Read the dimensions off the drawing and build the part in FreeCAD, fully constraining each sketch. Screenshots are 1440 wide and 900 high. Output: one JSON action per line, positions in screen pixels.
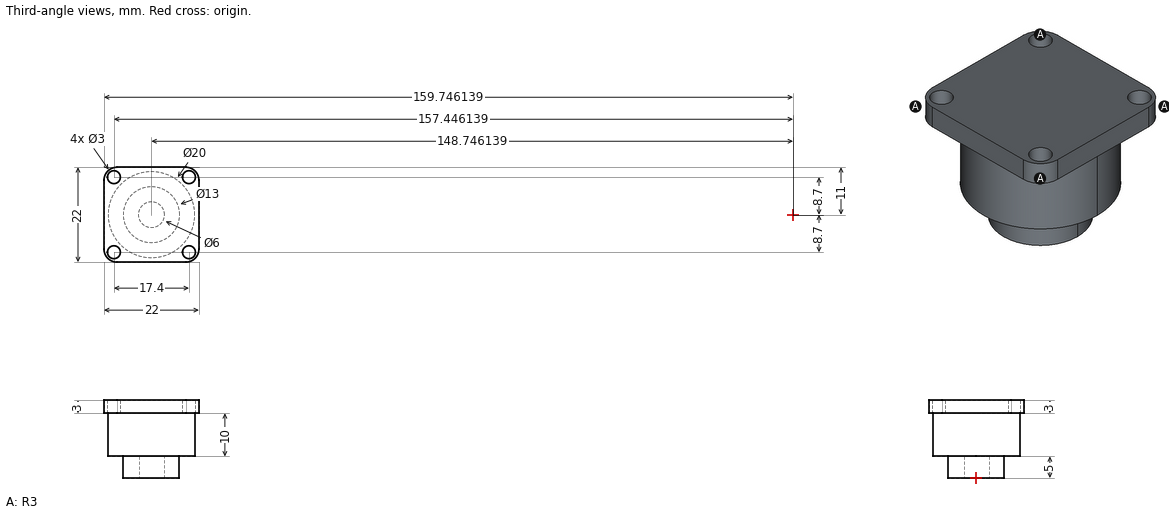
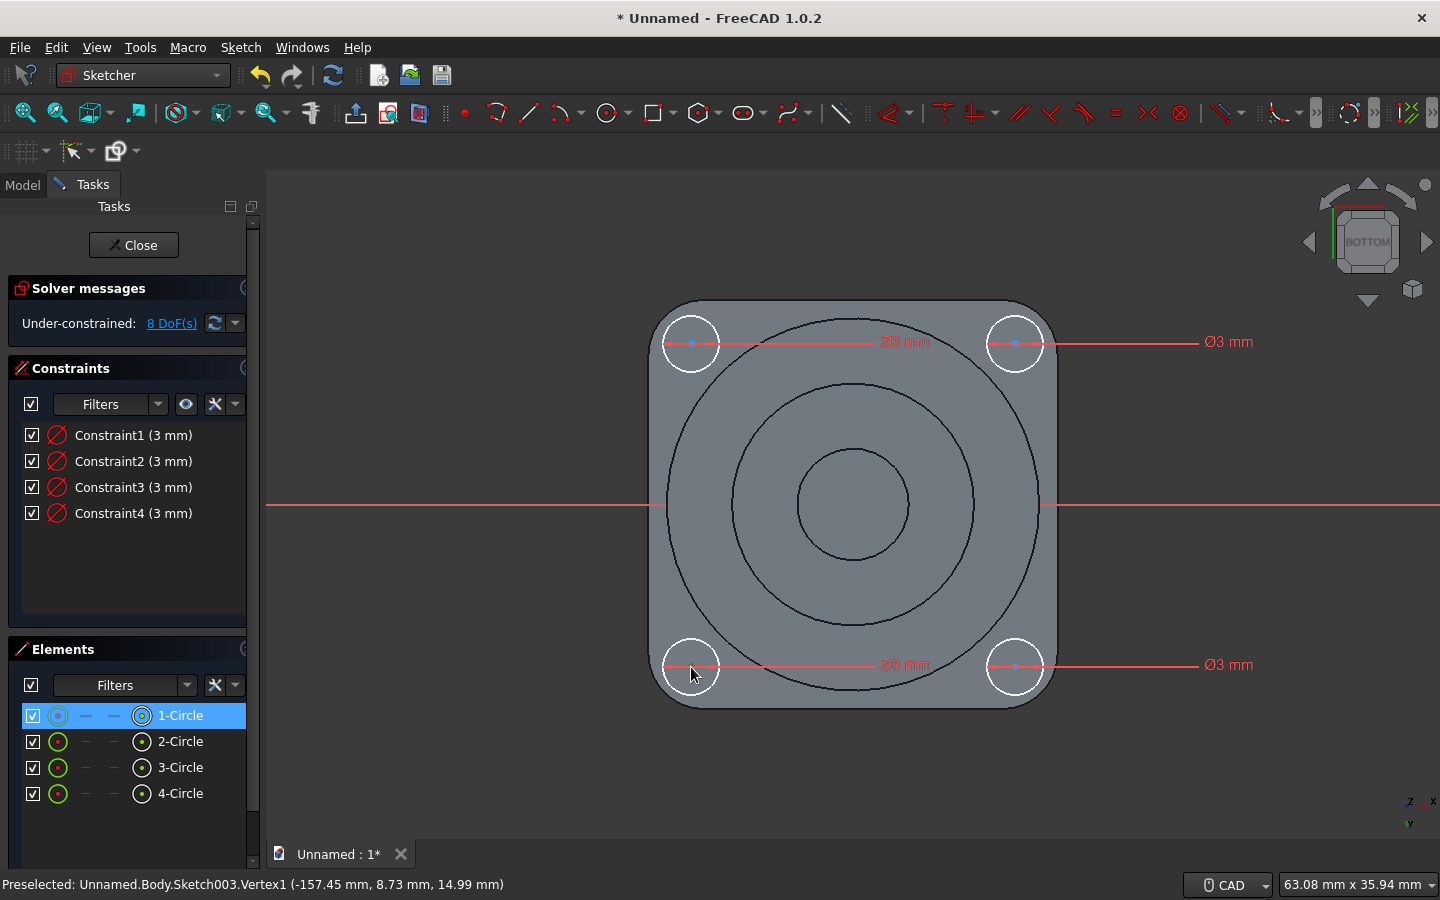
{"action": "left_click", "coordinate": [691, 344]}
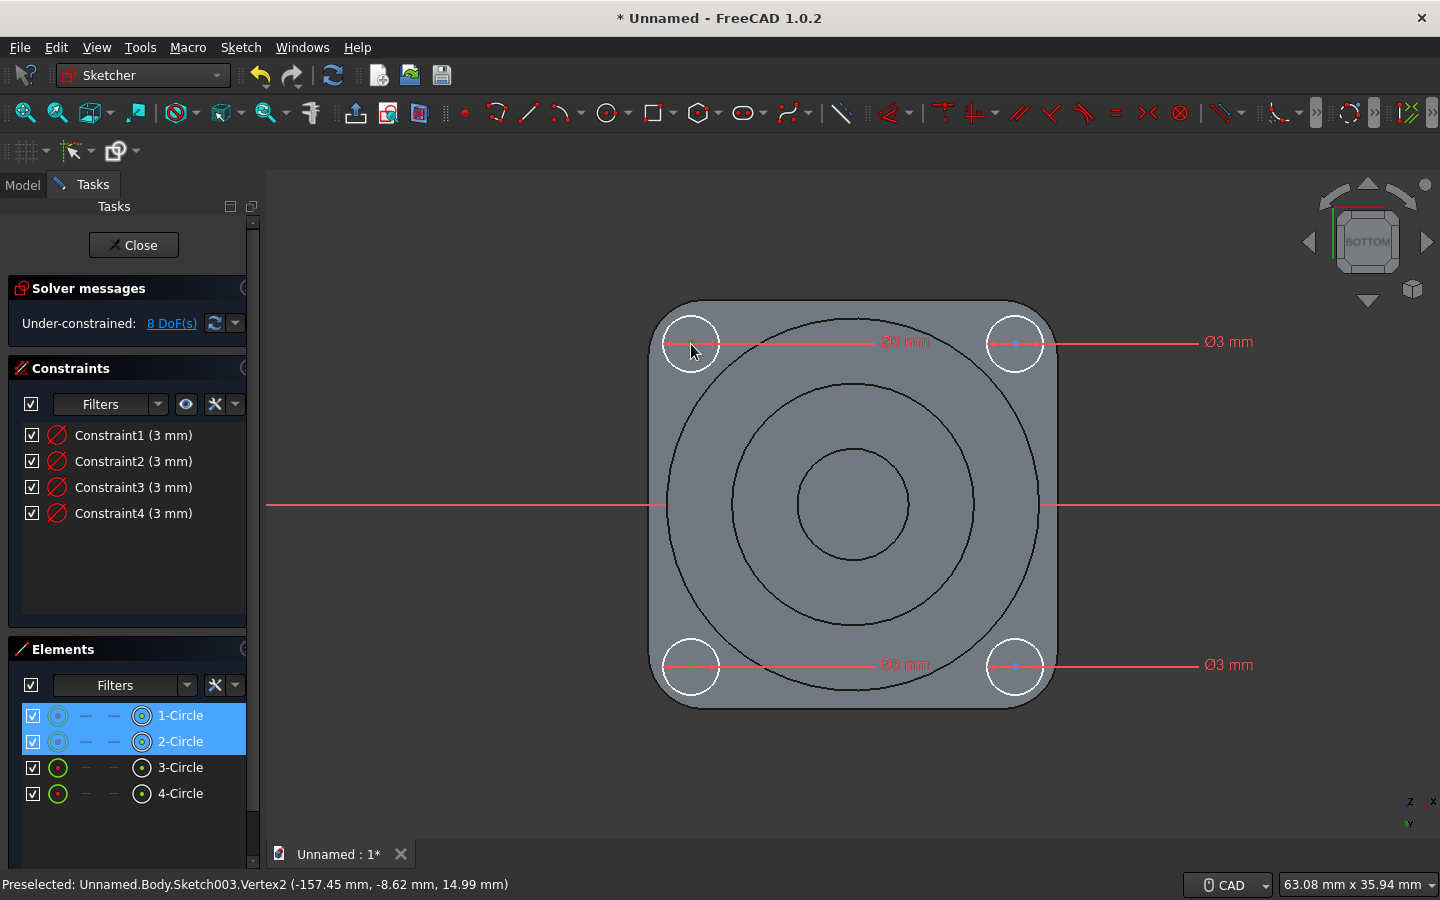
{"action": "key", "text": "v"}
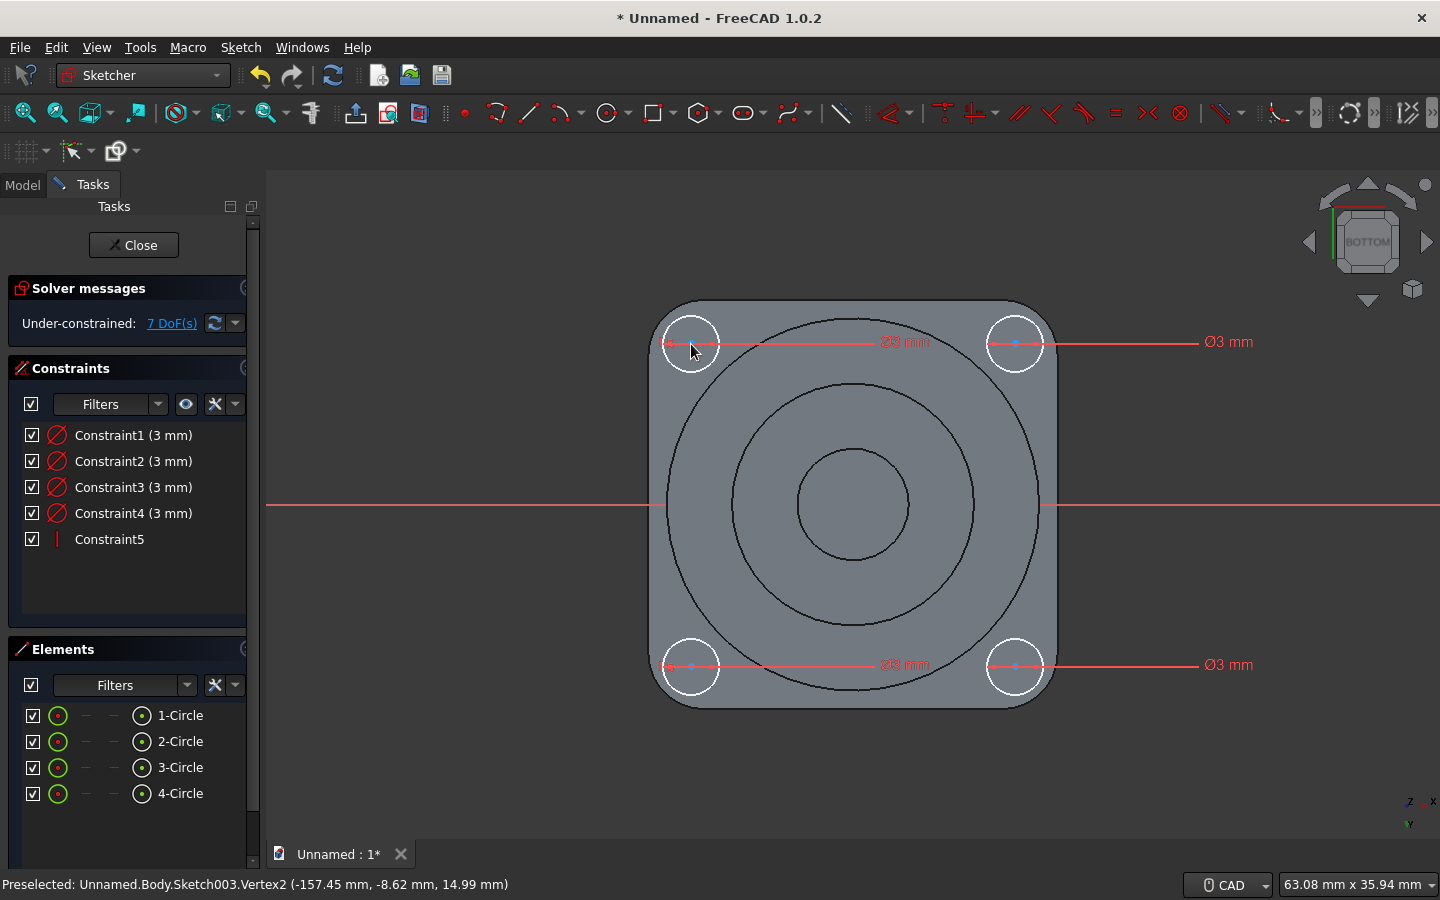
{"action": "left_click", "coordinate": [691, 344]}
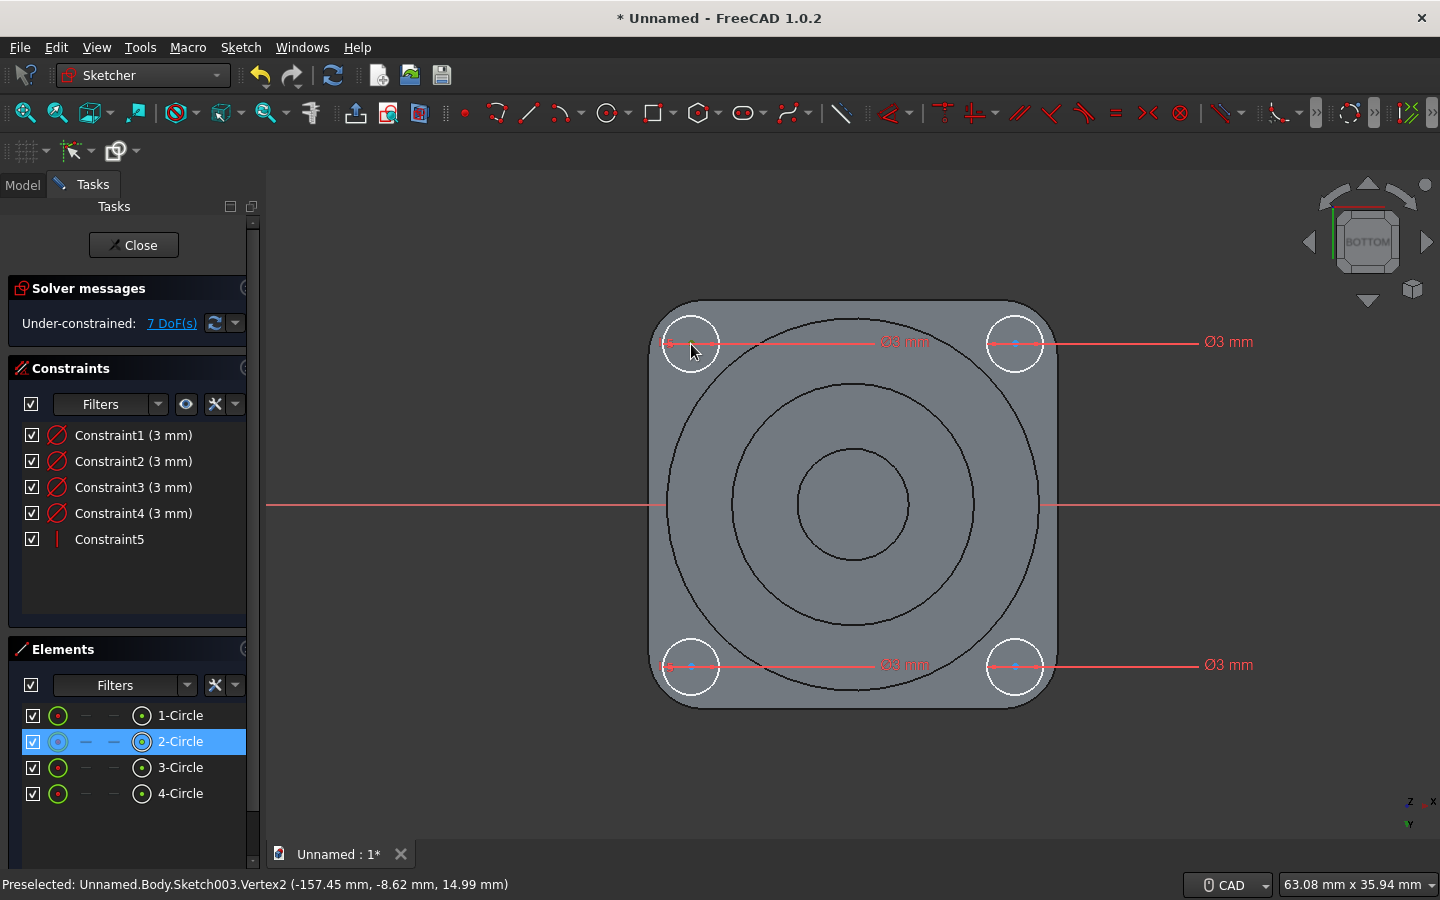
{"action": "left_click", "coordinate": [1015, 344]}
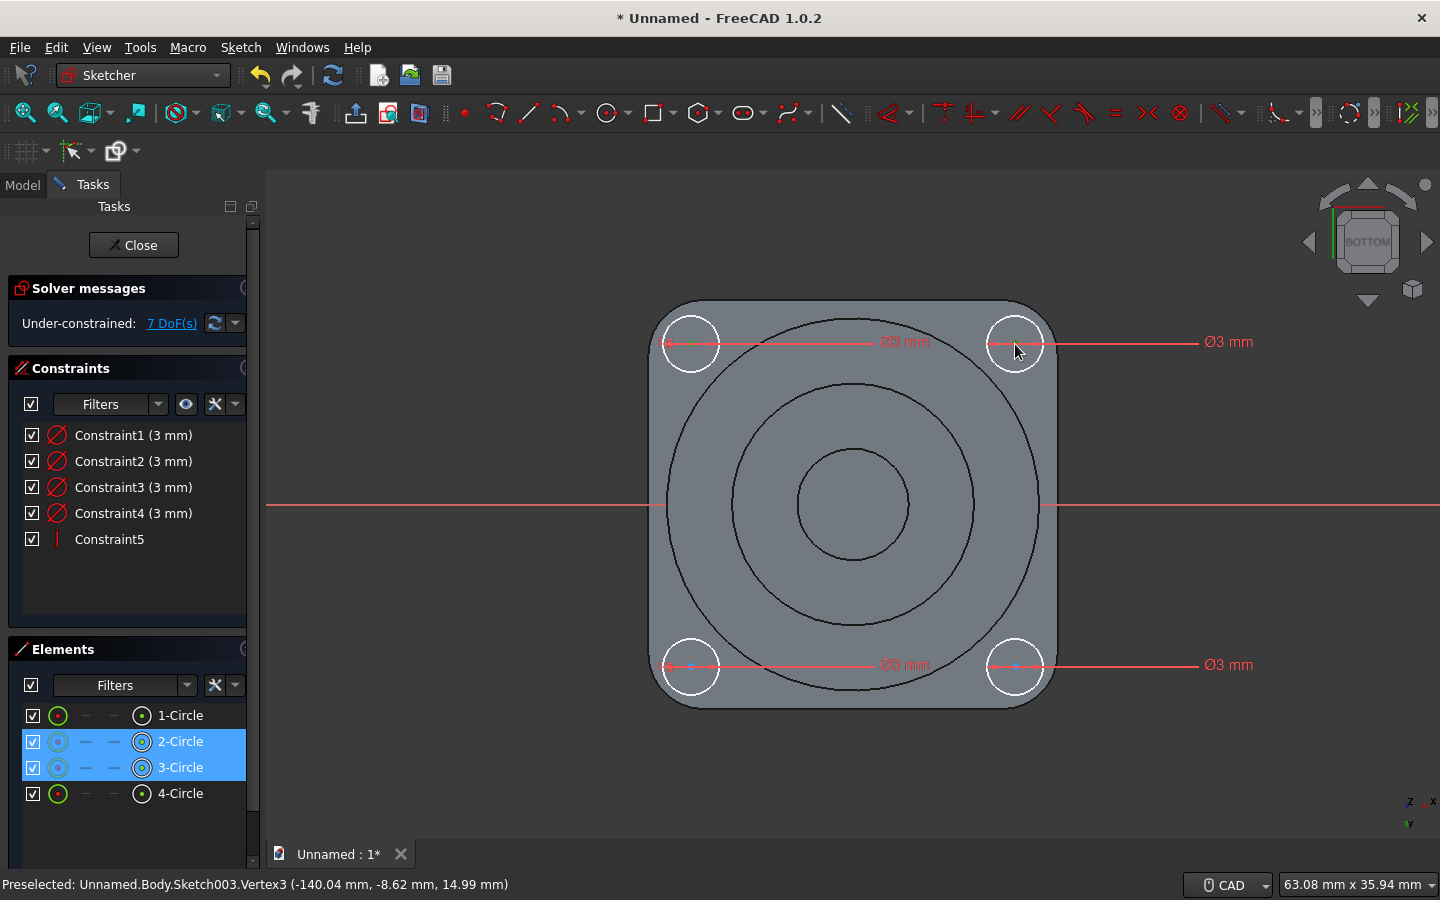
{"action": "left_click", "coordinate": [998, 114]}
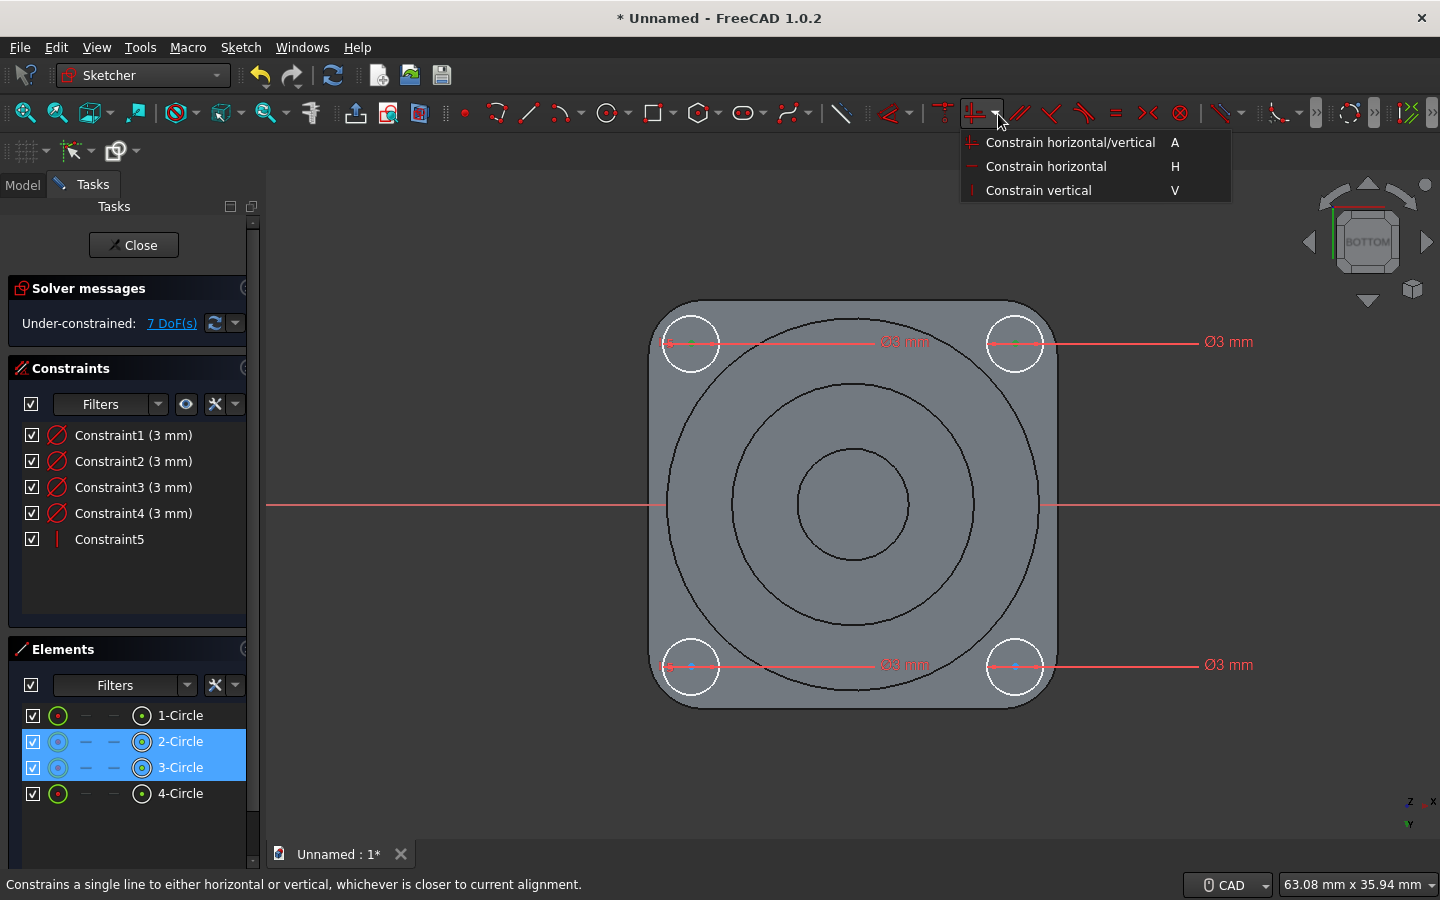
{"action": "left_click", "coordinate": [1096, 166]}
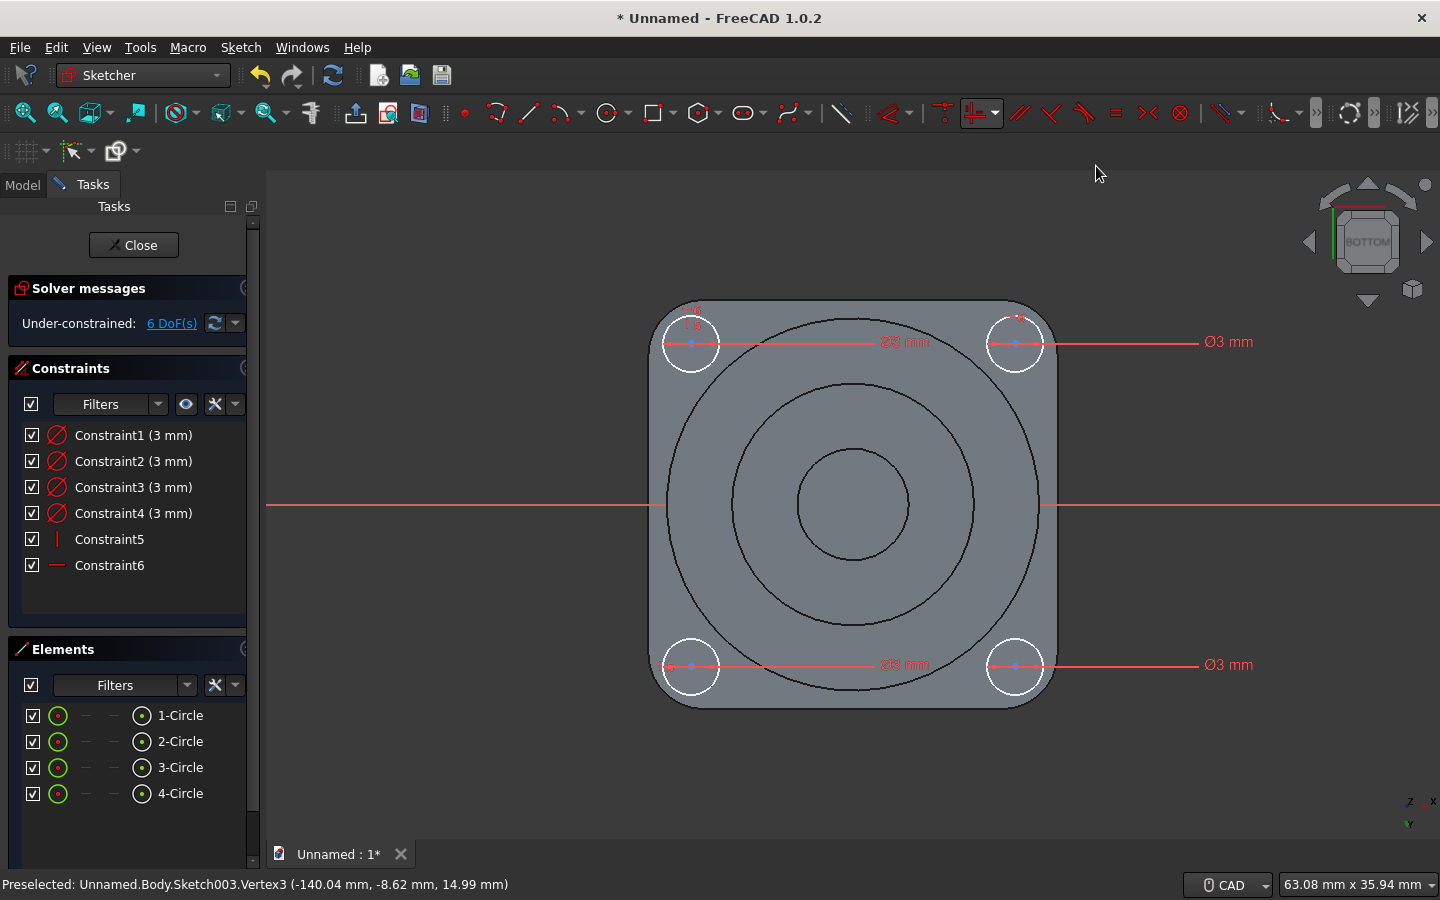
{"action": "left_click", "coordinate": [1015, 344]}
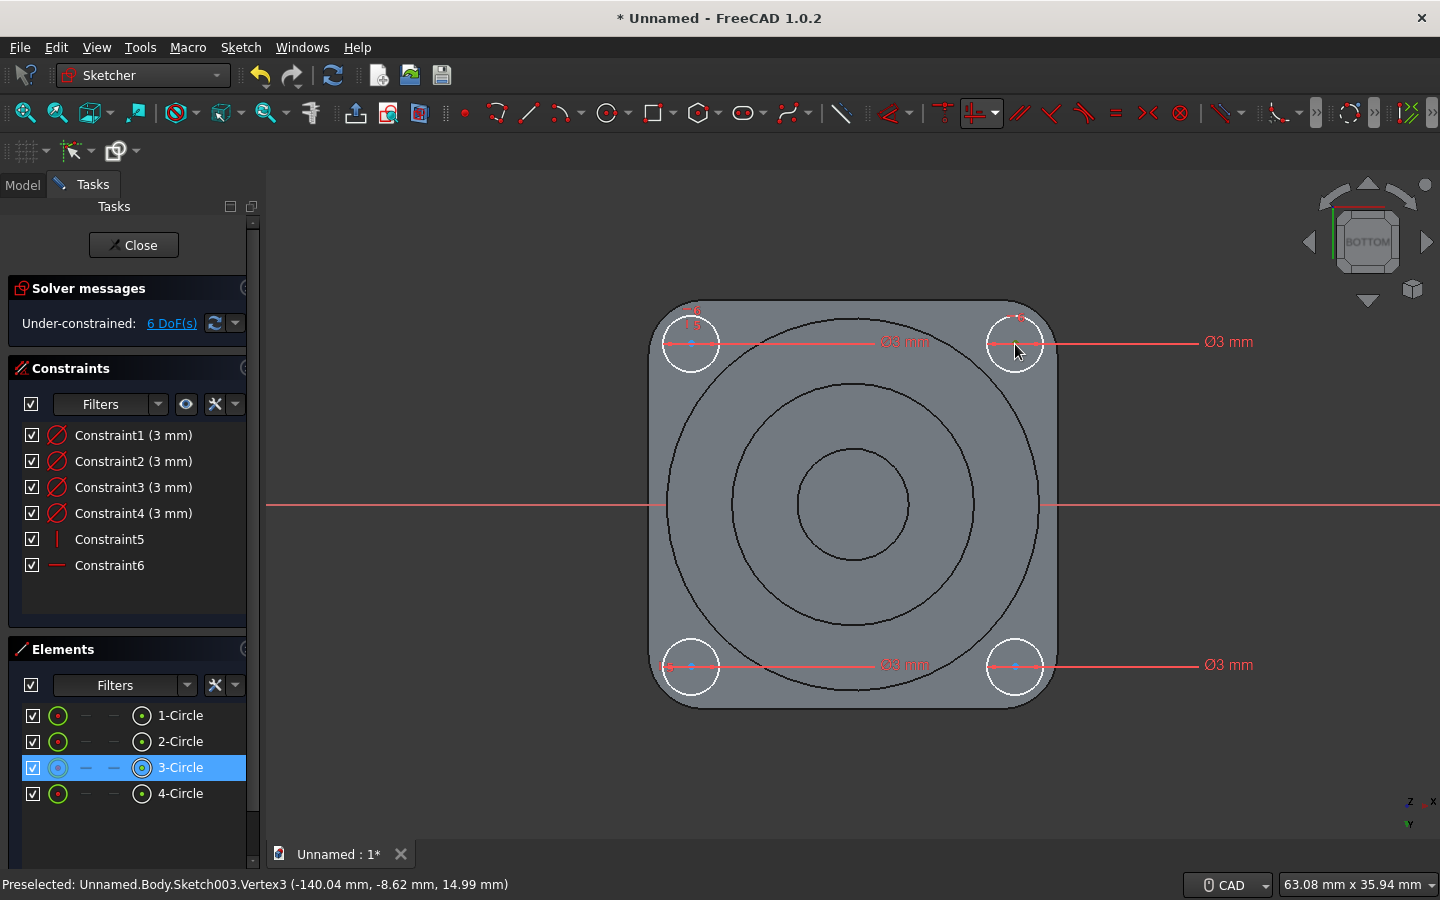
{"action": "left_click", "coordinate": [1015, 667]}